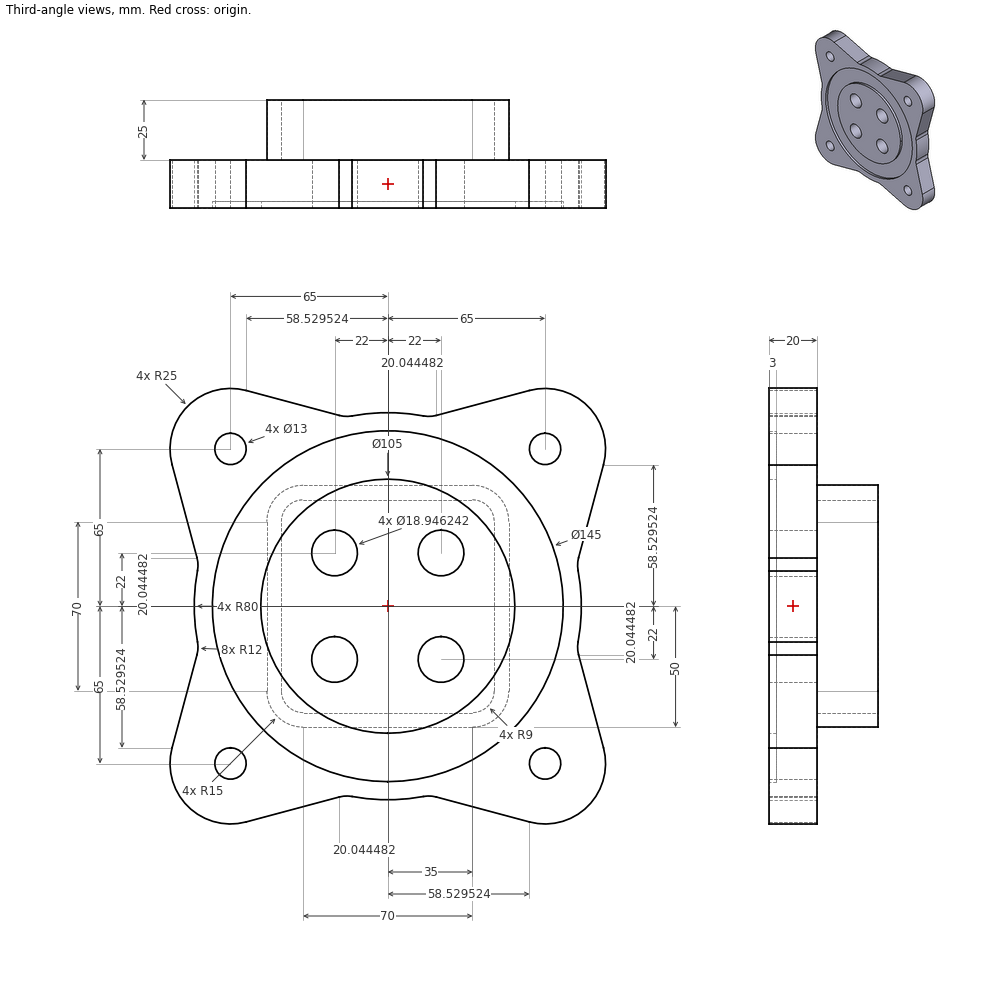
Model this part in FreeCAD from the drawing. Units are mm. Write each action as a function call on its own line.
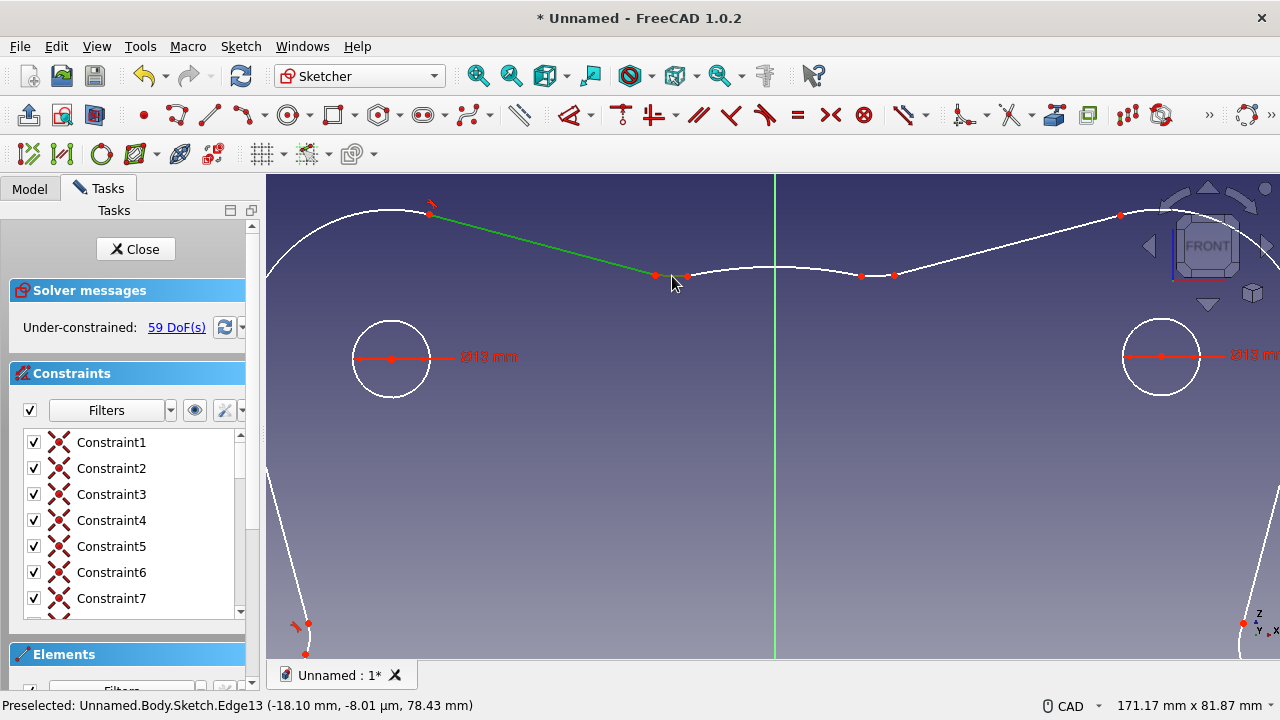
key(t)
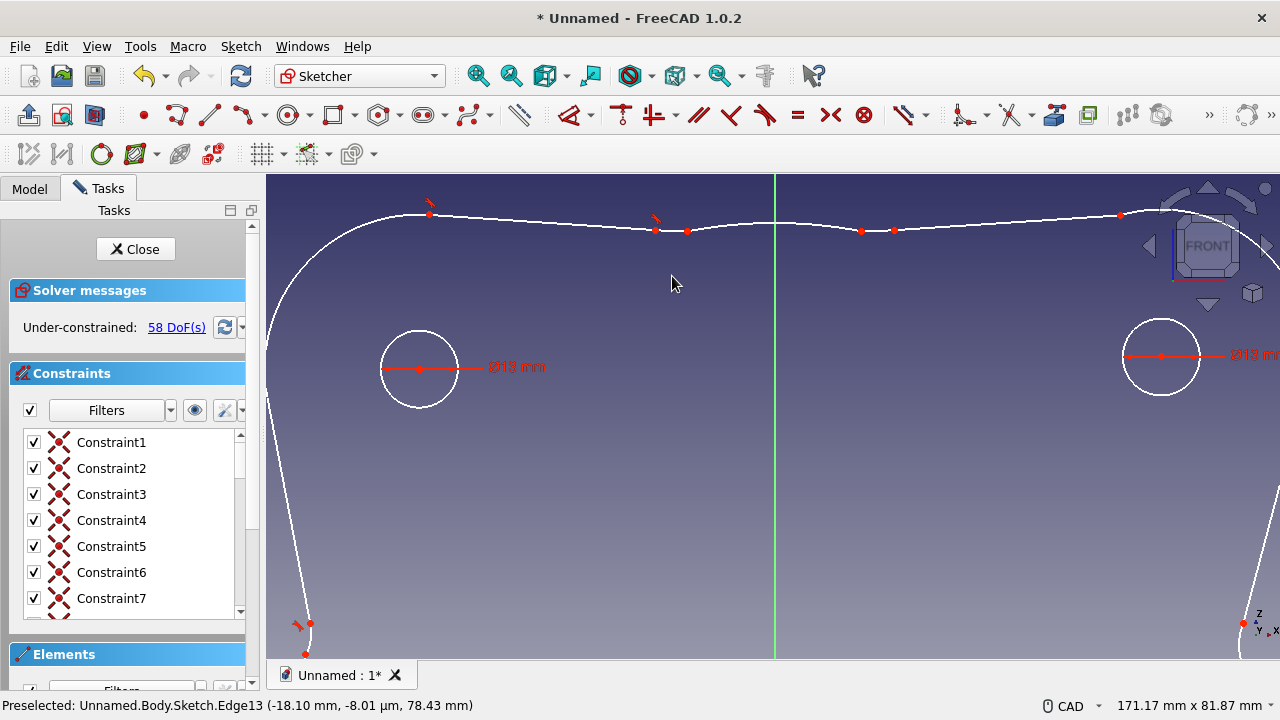
click(962, 226)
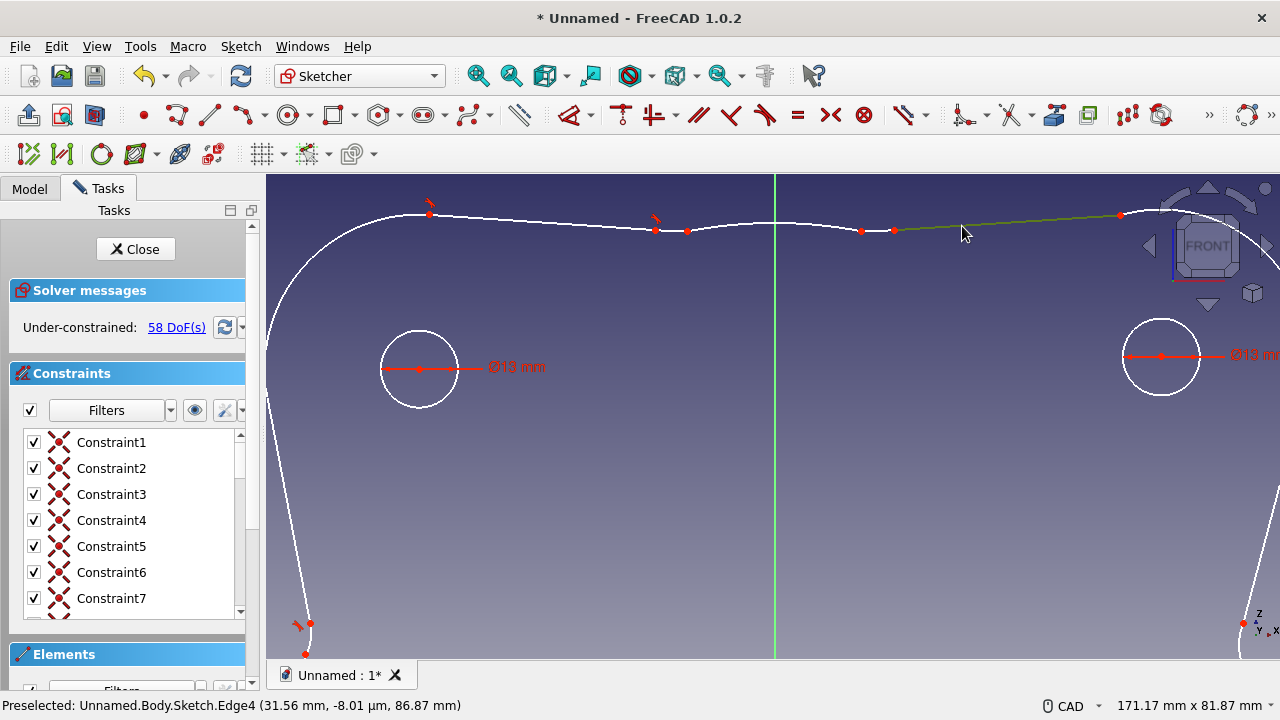
scroll(871, 231, up, 2)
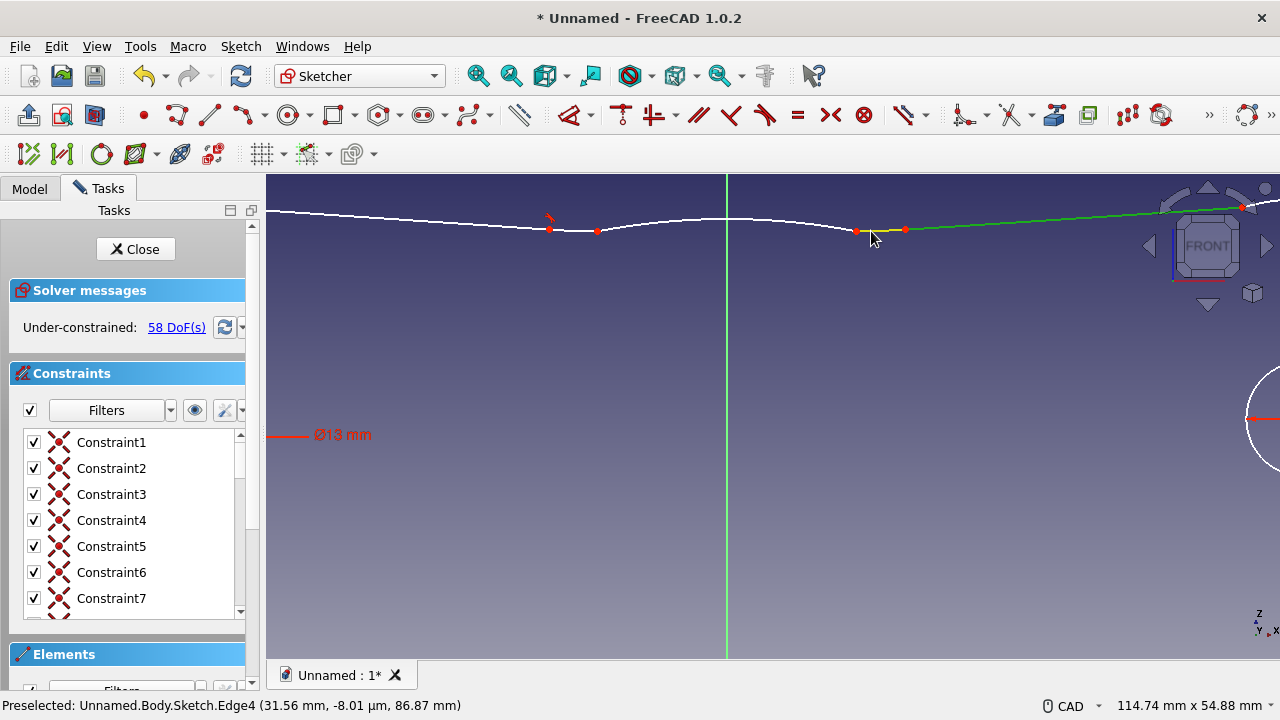
click(871, 231)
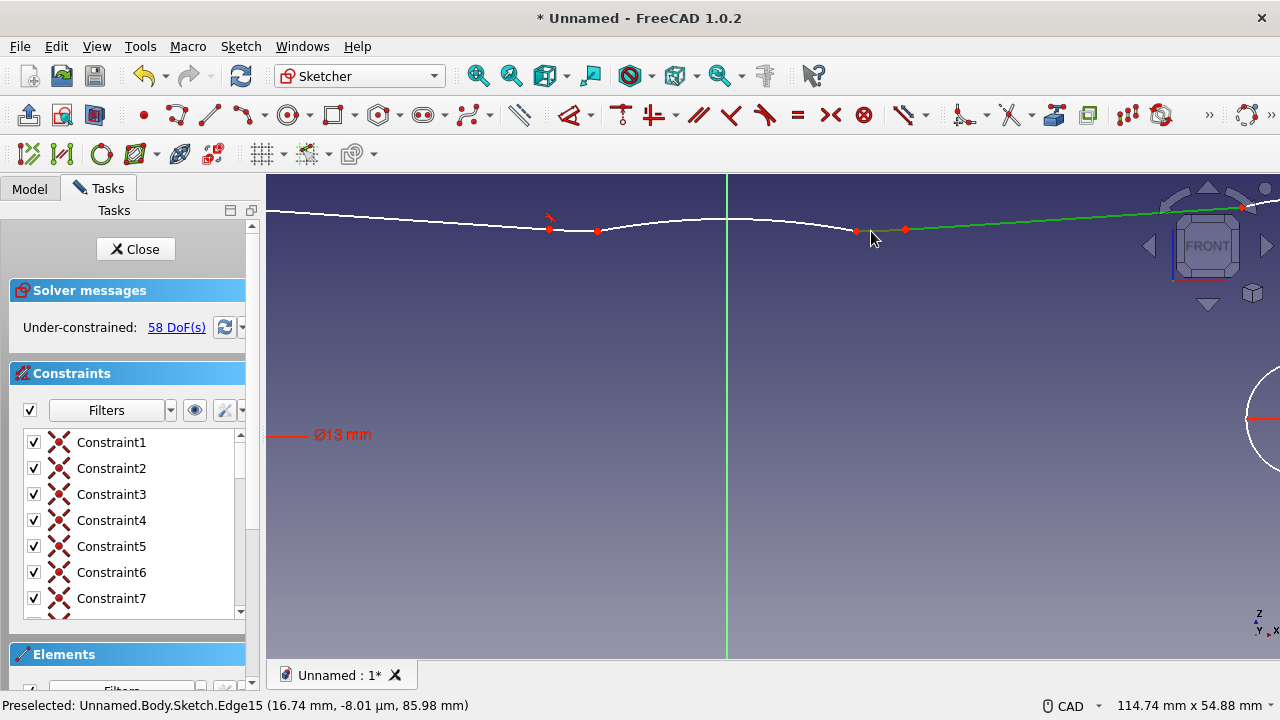
click(765, 116)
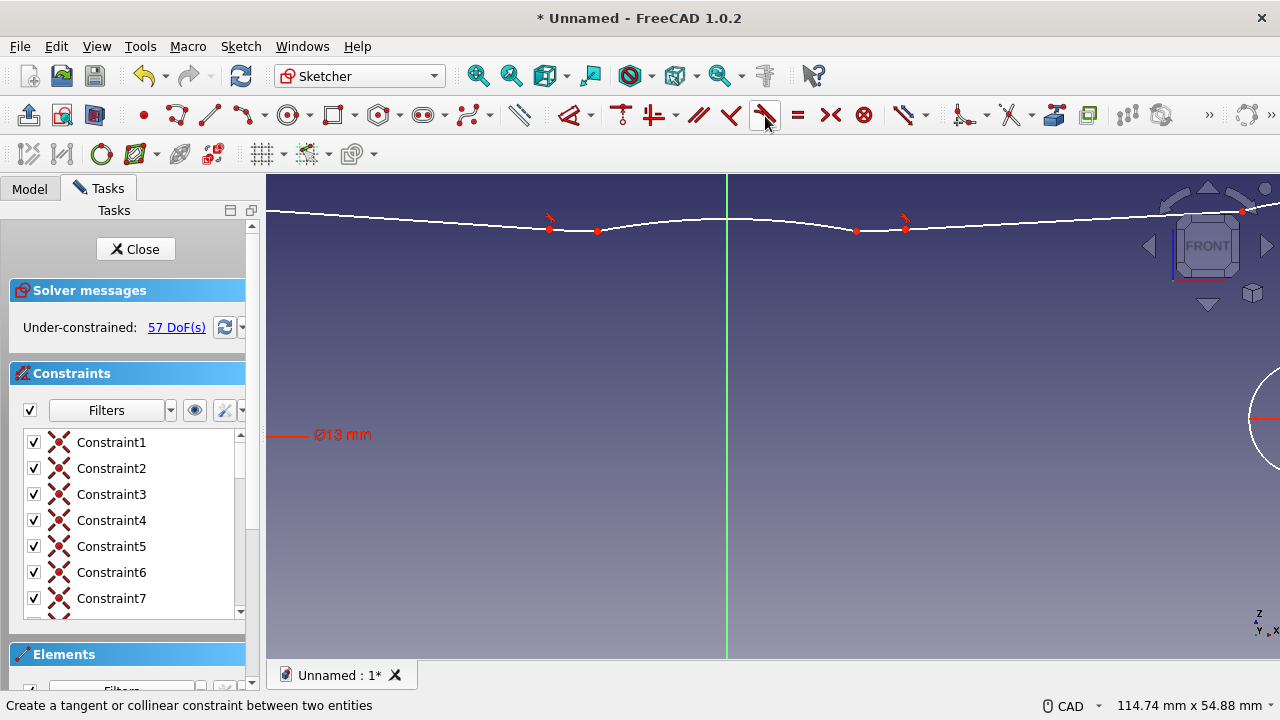
scroll(699, 271, down, 8)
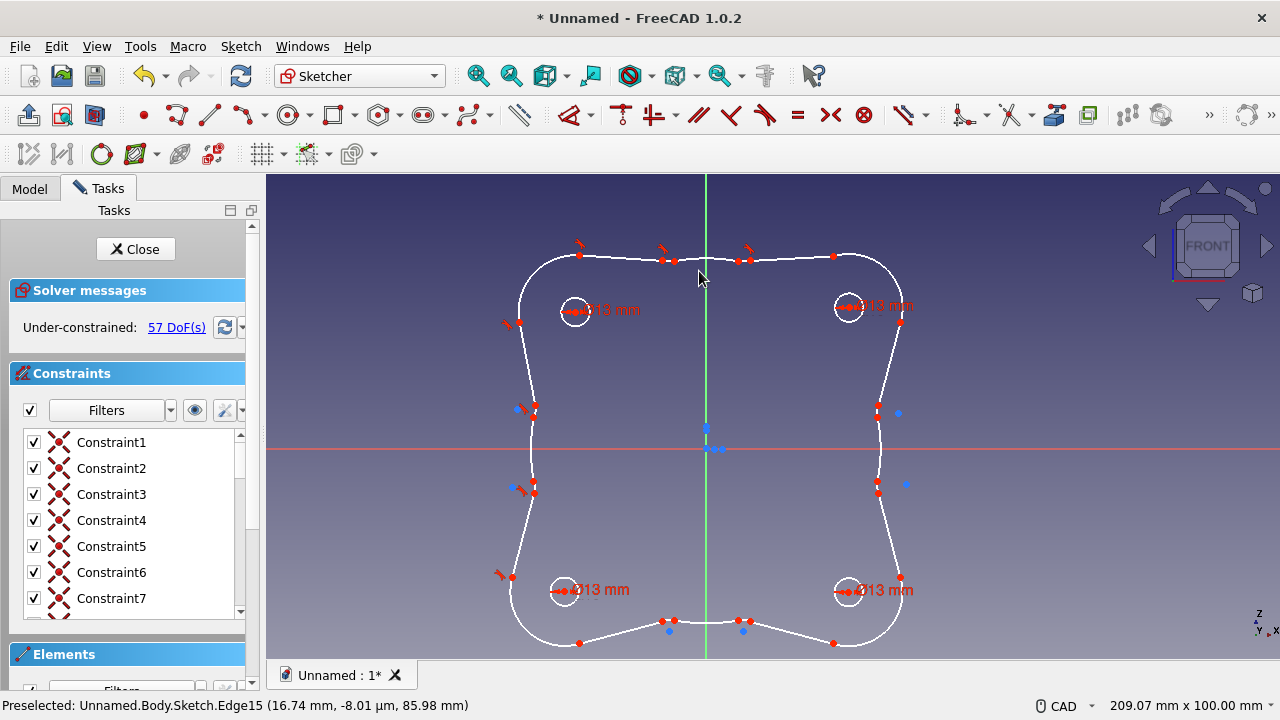
click(762, 262)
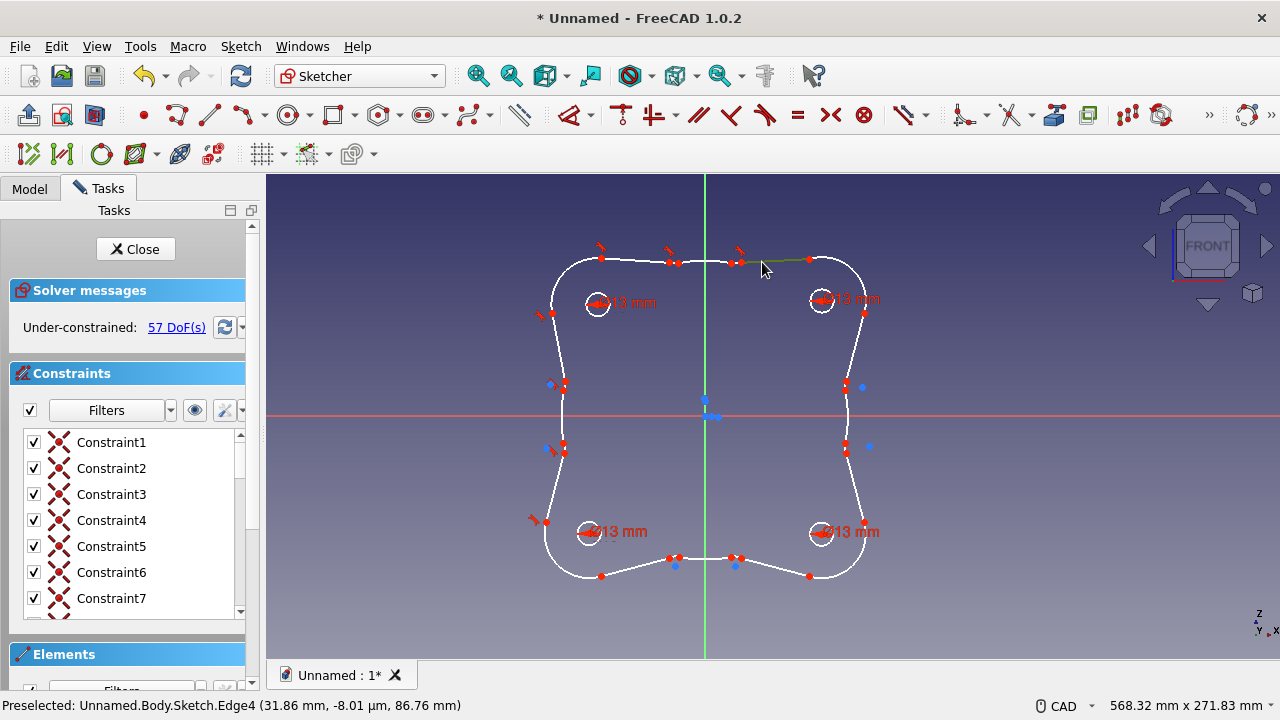
click(863, 286)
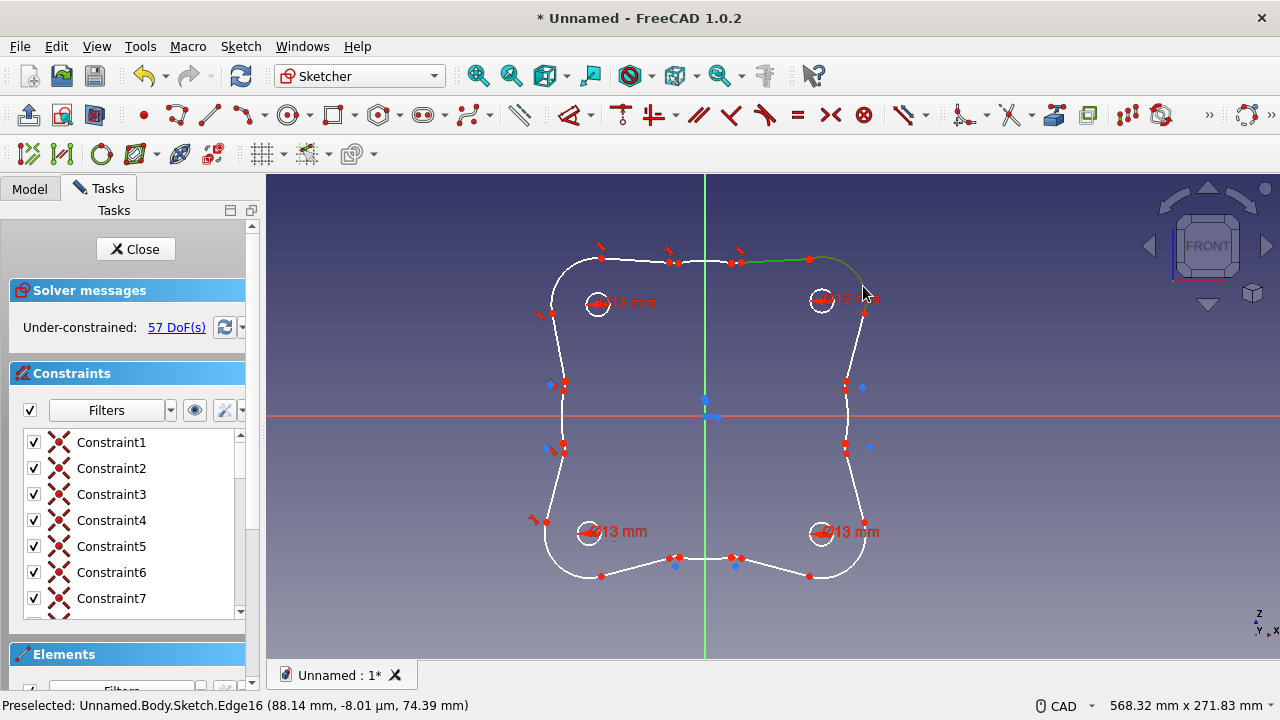
click(765, 116)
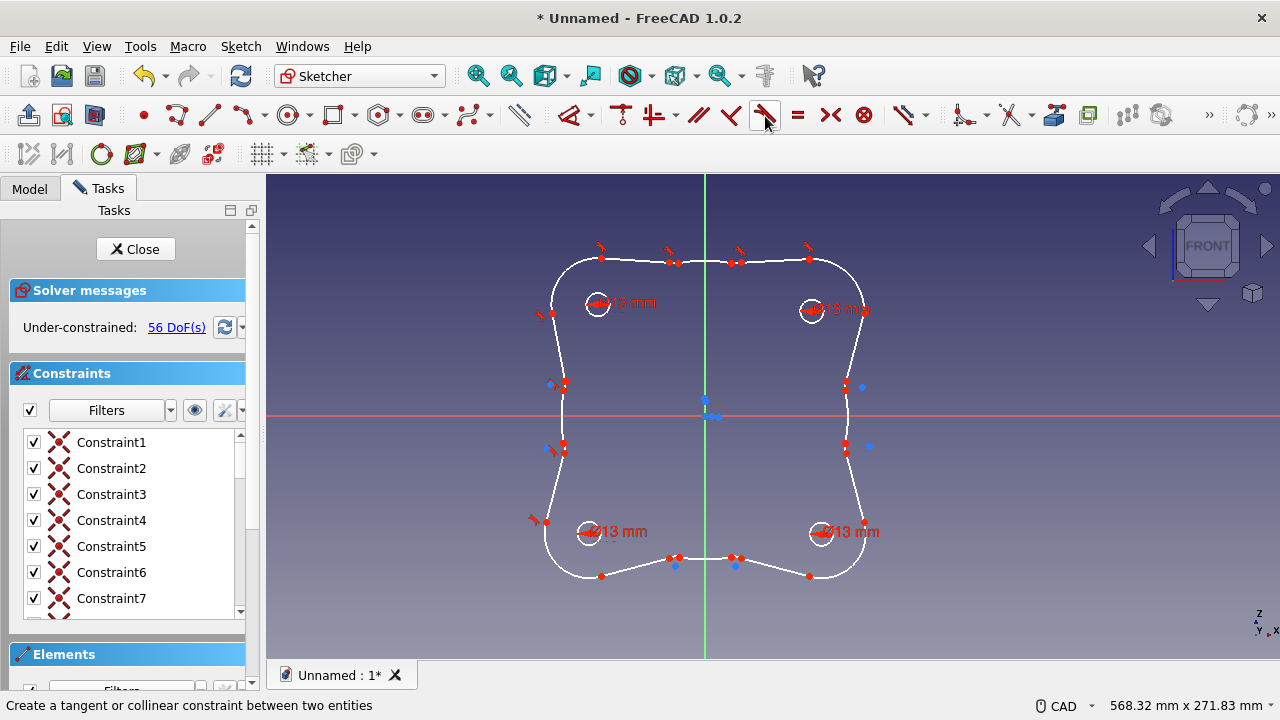
click(859, 334)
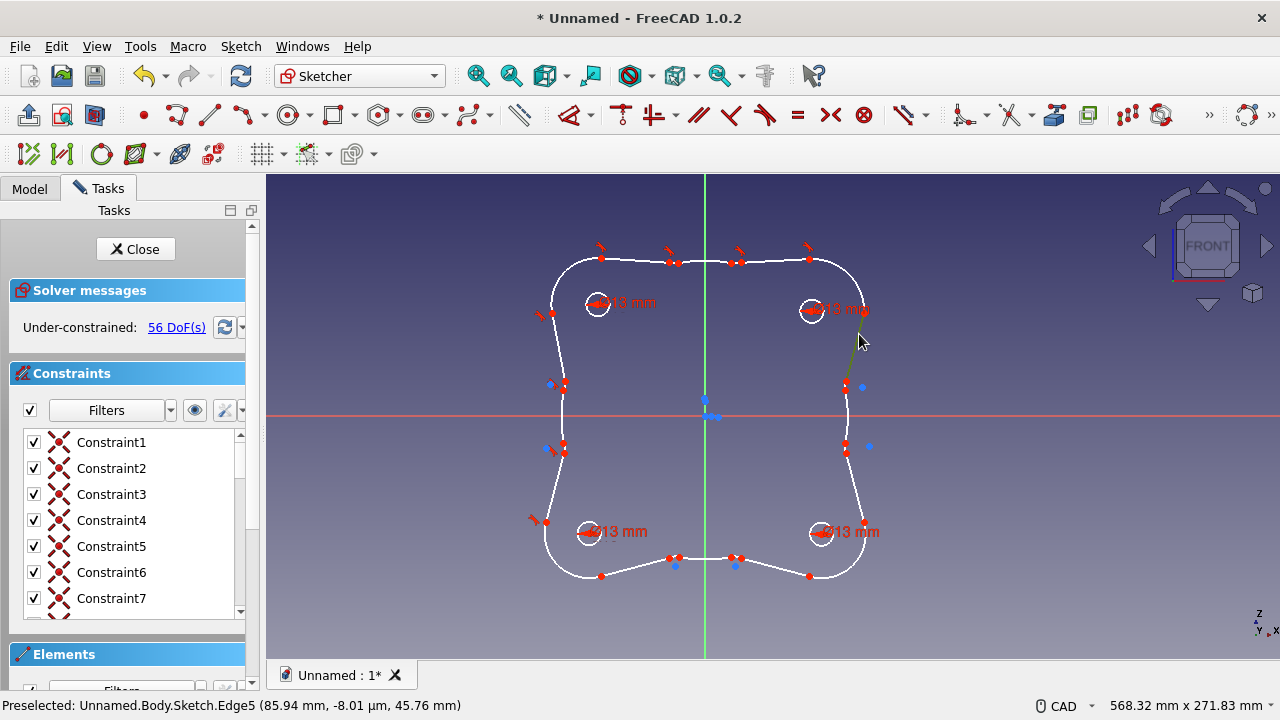
click(859, 288)